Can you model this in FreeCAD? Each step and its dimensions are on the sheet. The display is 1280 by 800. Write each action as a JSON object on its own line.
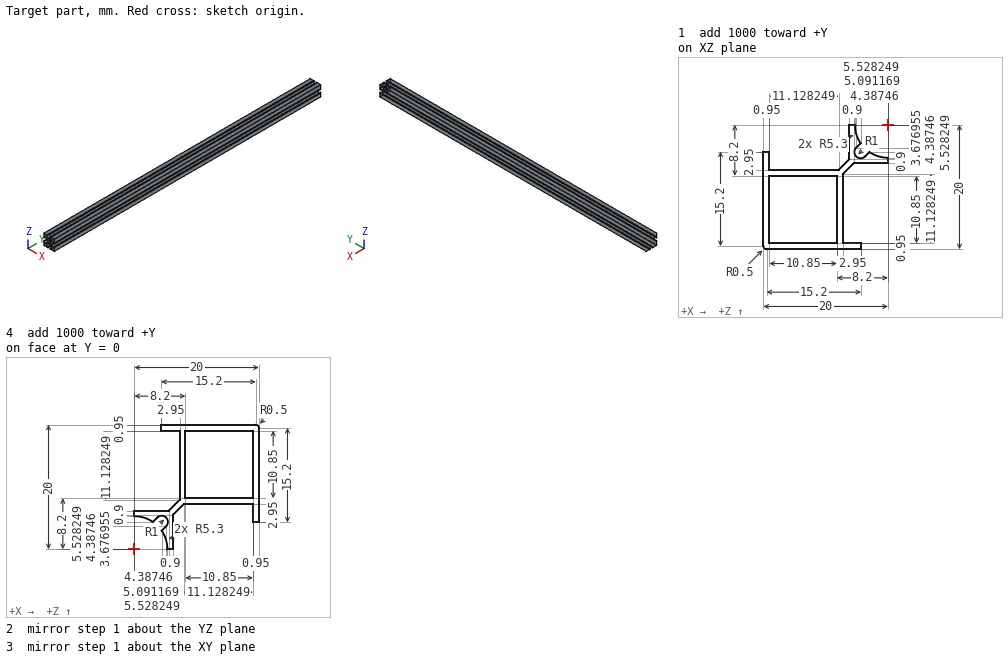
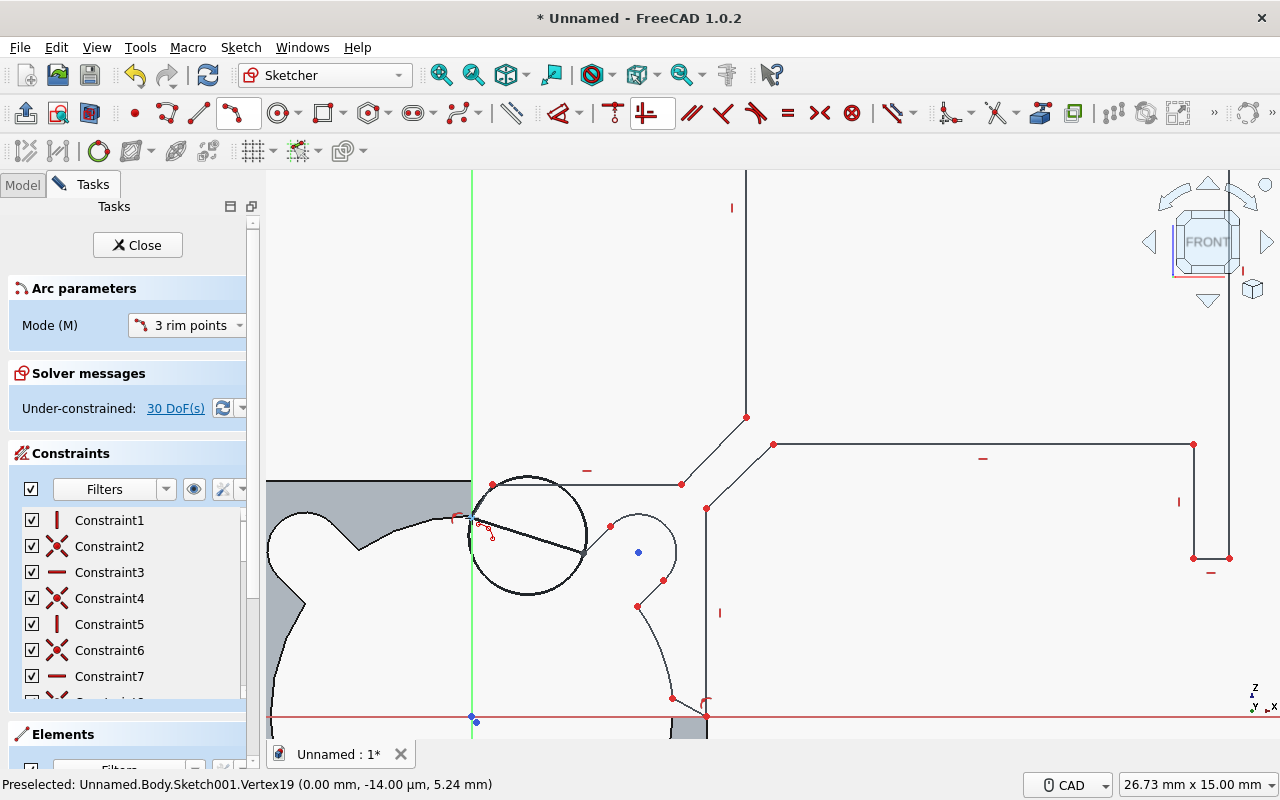
{"action": "scroll", "coordinate": [531, 524], "scroll_direction": "up", "scroll_amount": 3}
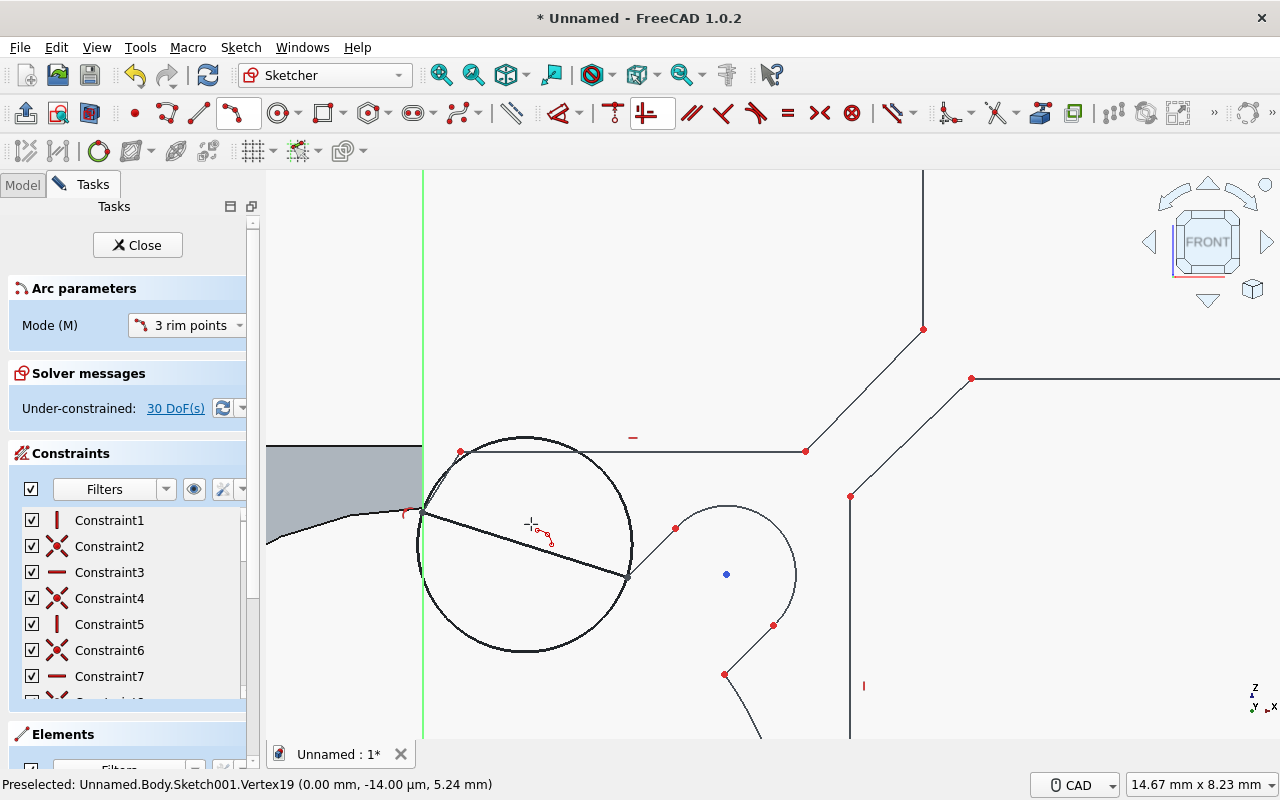
{"action": "left_click", "coordinate": [530, 524]}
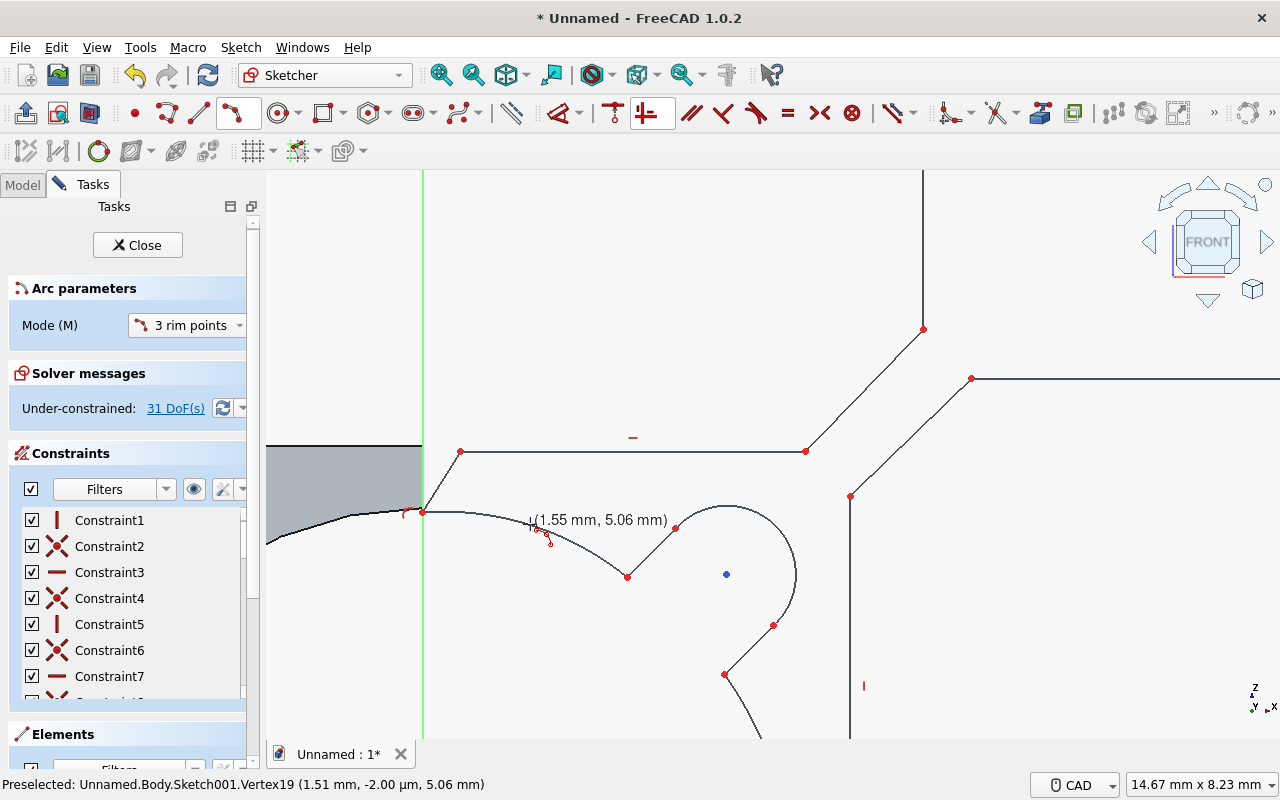
{"action": "scroll", "coordinate": [571, 543], "scroll_direction": "down", "scroll_amount": 7}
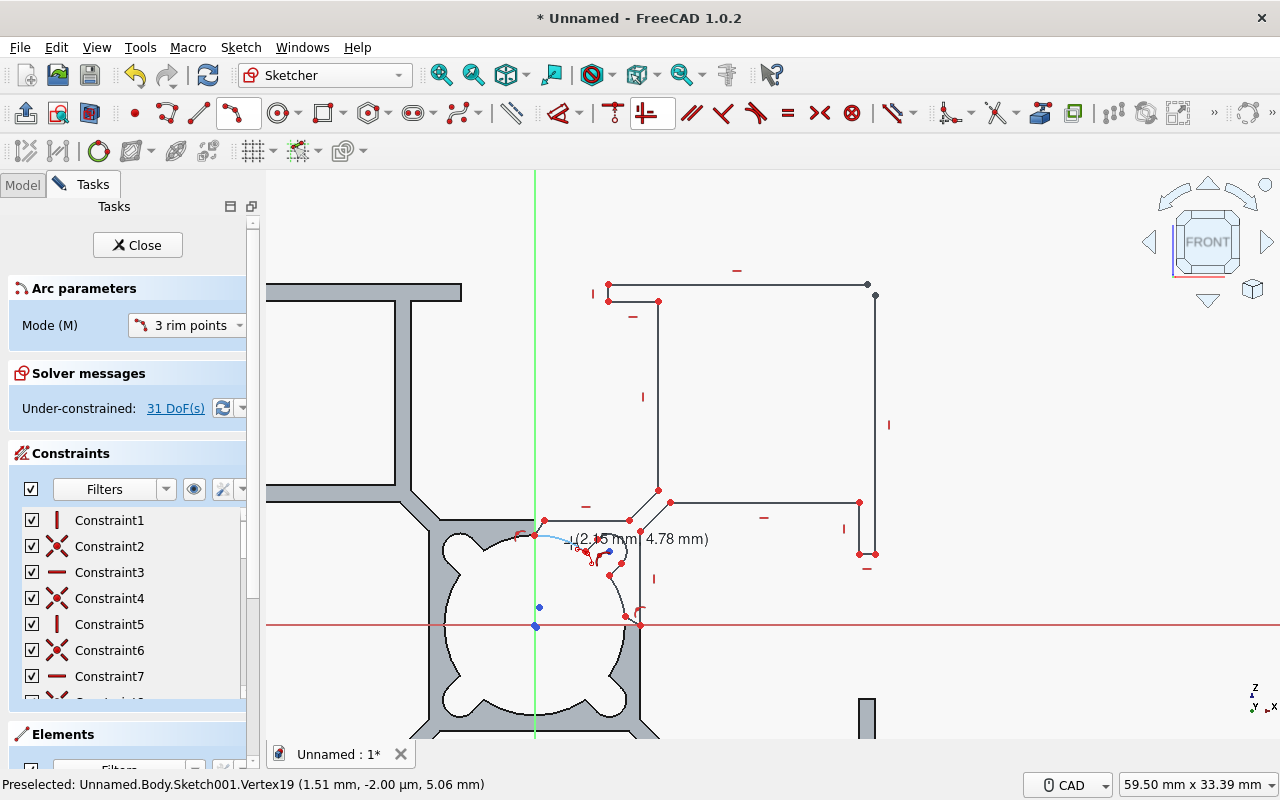
{"action": "scroll", "coordinate": [867, 284], "scroll_direction": "up", "scroll_amount": 2}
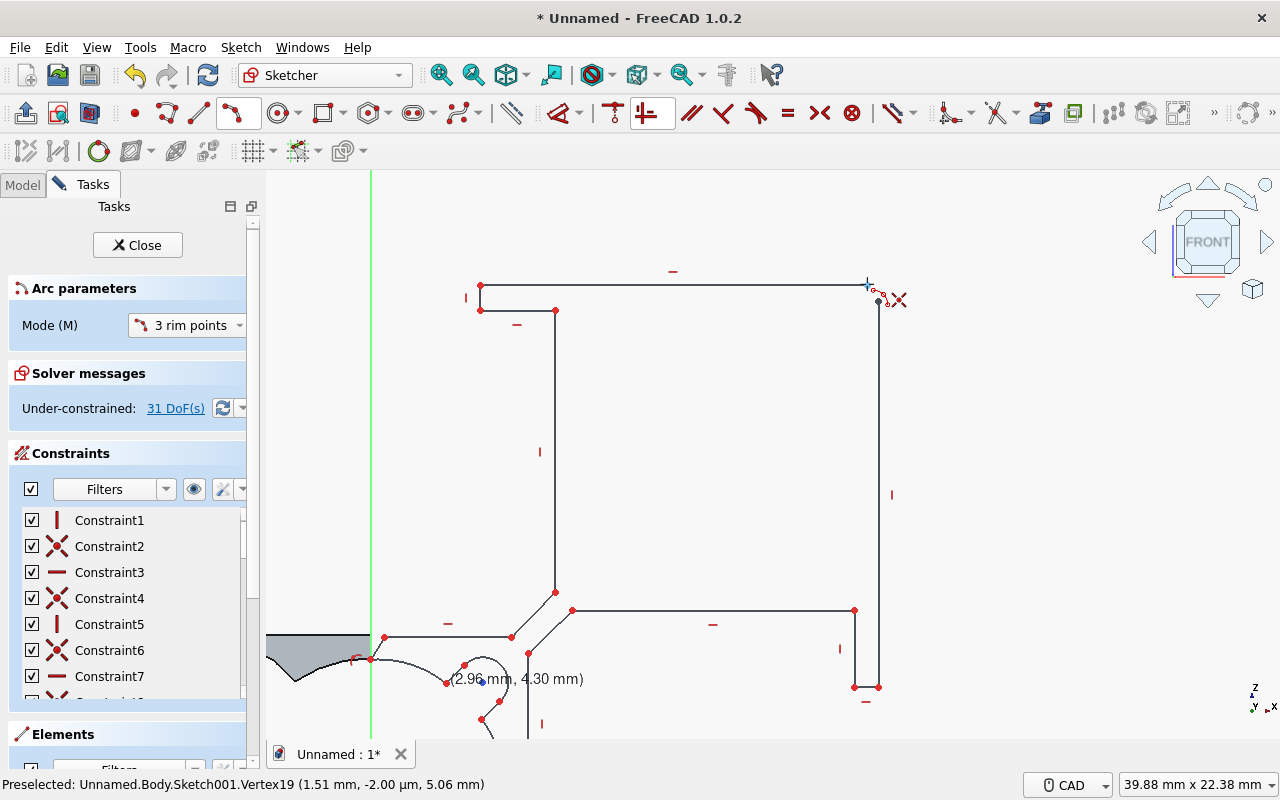
{"action": "left_click", "coordinate": [867, 285]}
{"action": "left_click", "coordinate": [879, 301]}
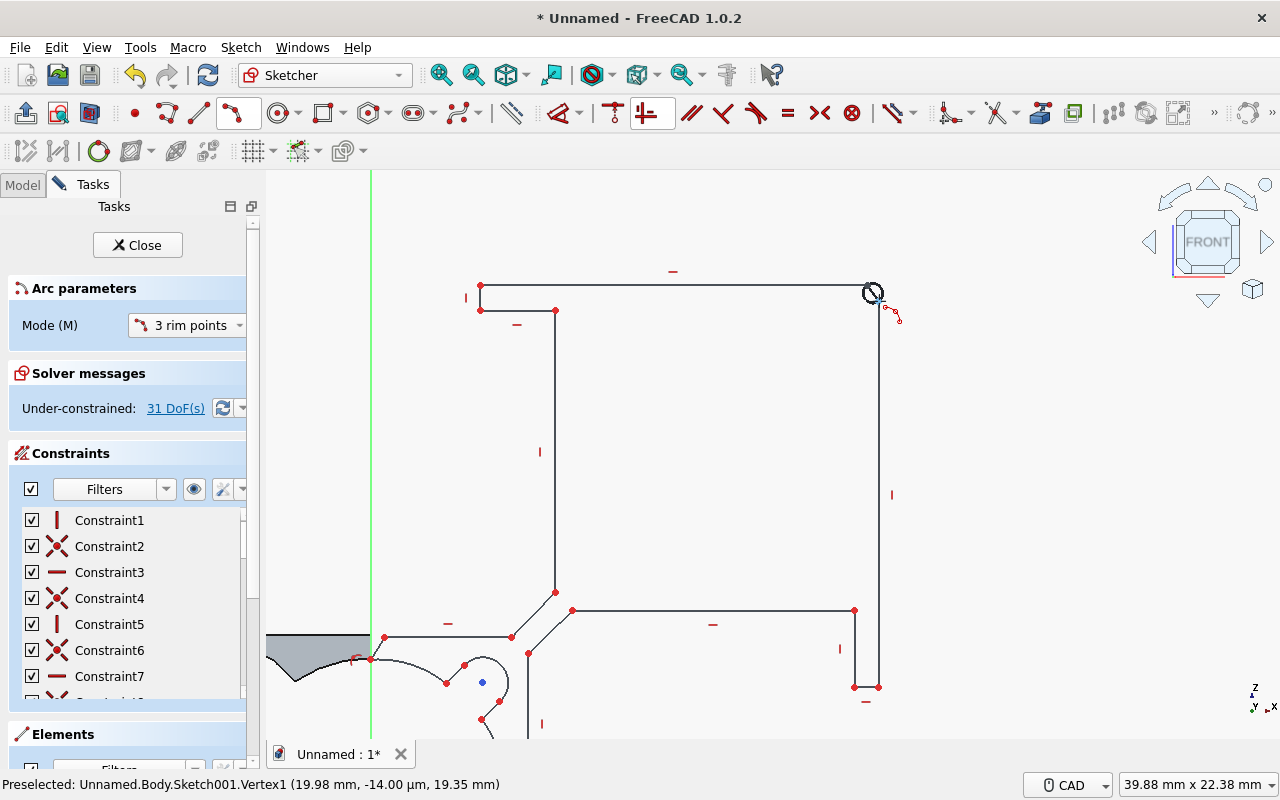
{"action": "scroll", "coordinate": [876, 288], "scroll_direction": "up", "scroll_amount": 8}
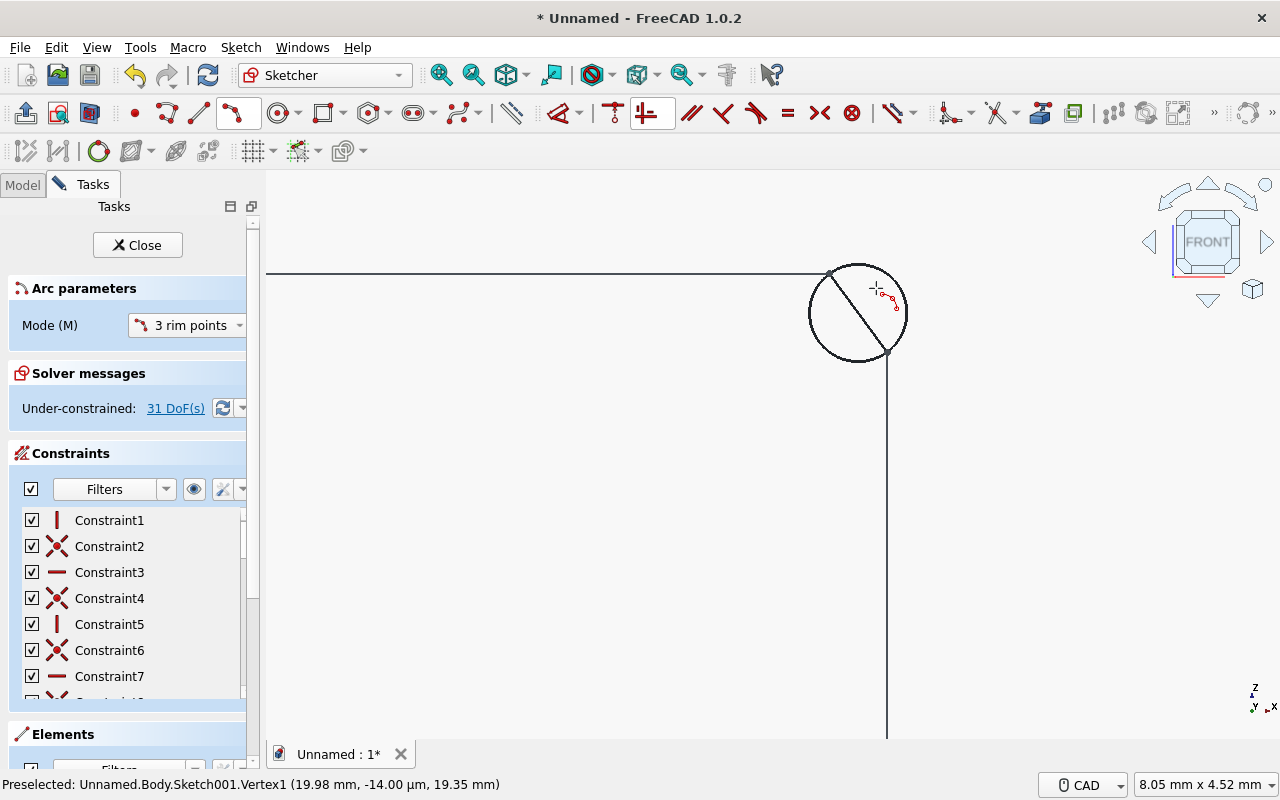
{"action": "left_click", "coordinate": [872, 288]}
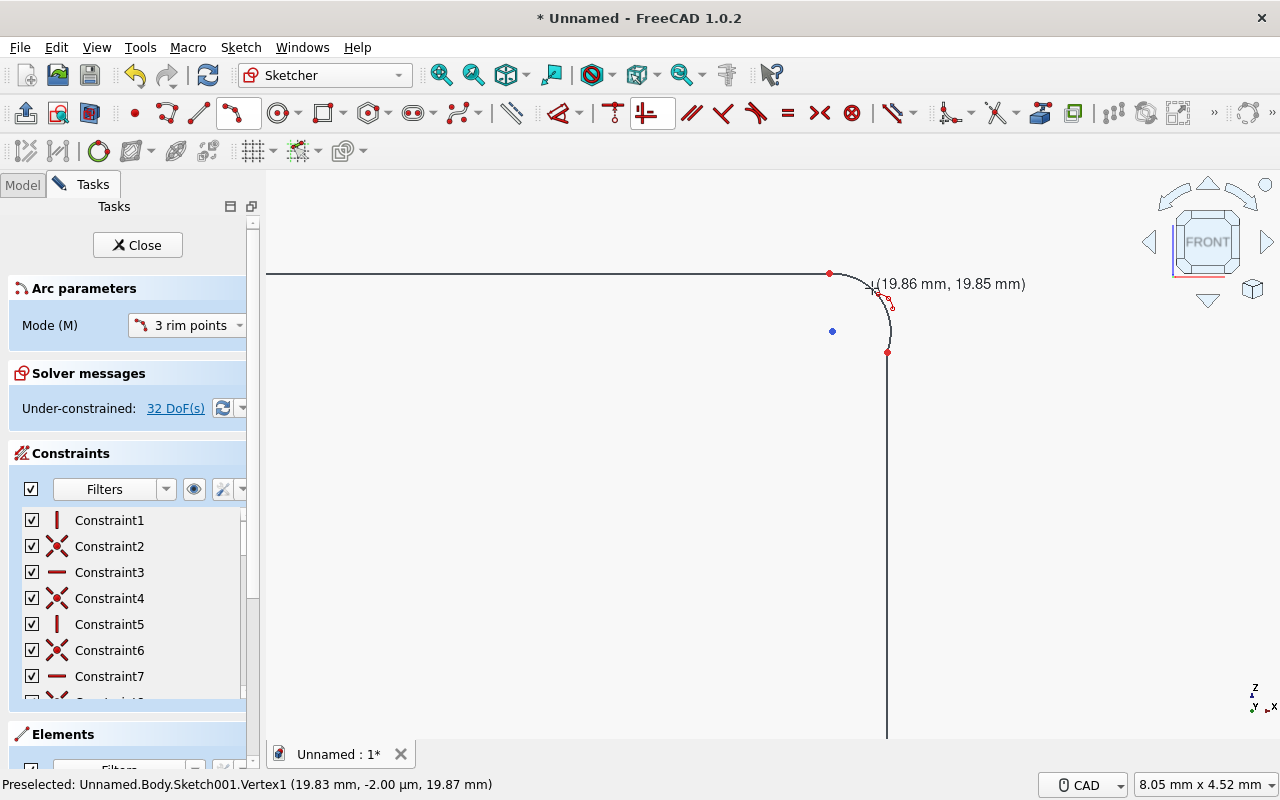
{"action": "key", "text": "g r"}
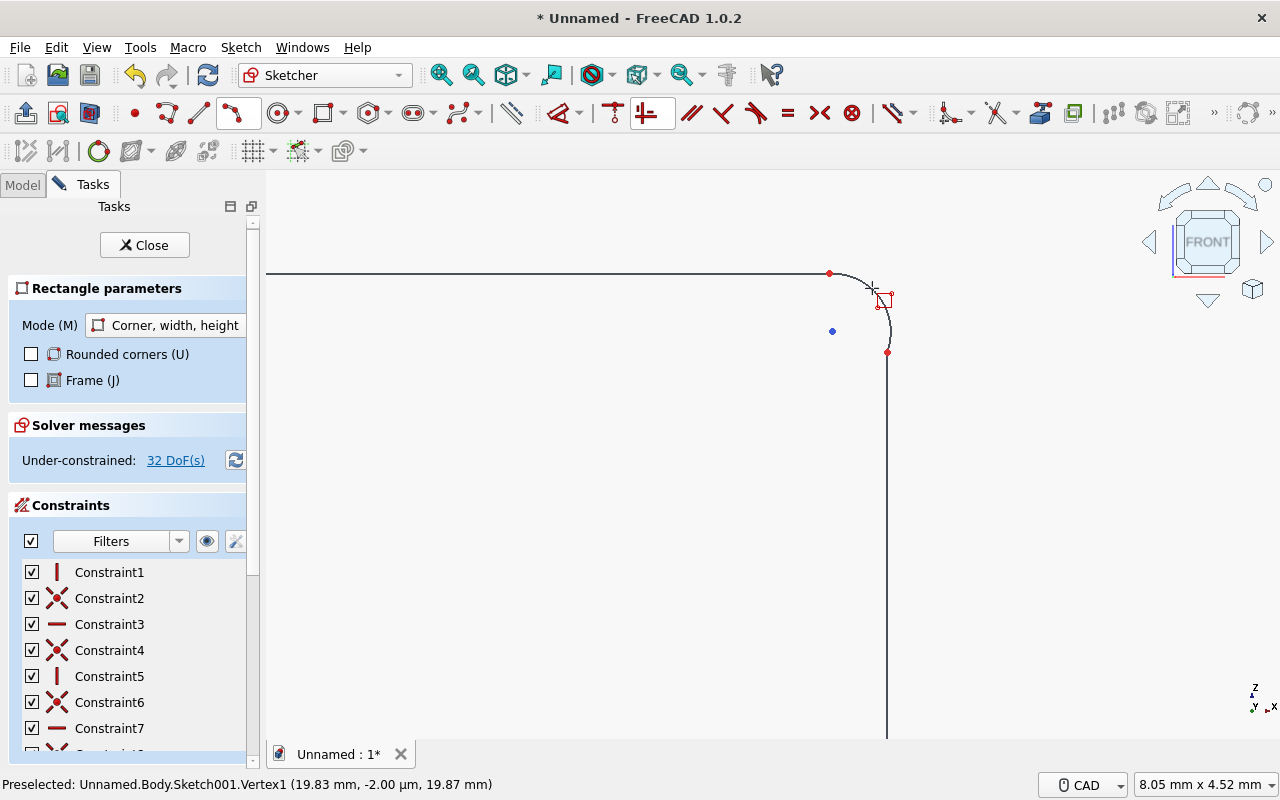
{"action": "scroll", "coordinate": [873, 286], "scroll_direction": "down", "scroll_amount": 10}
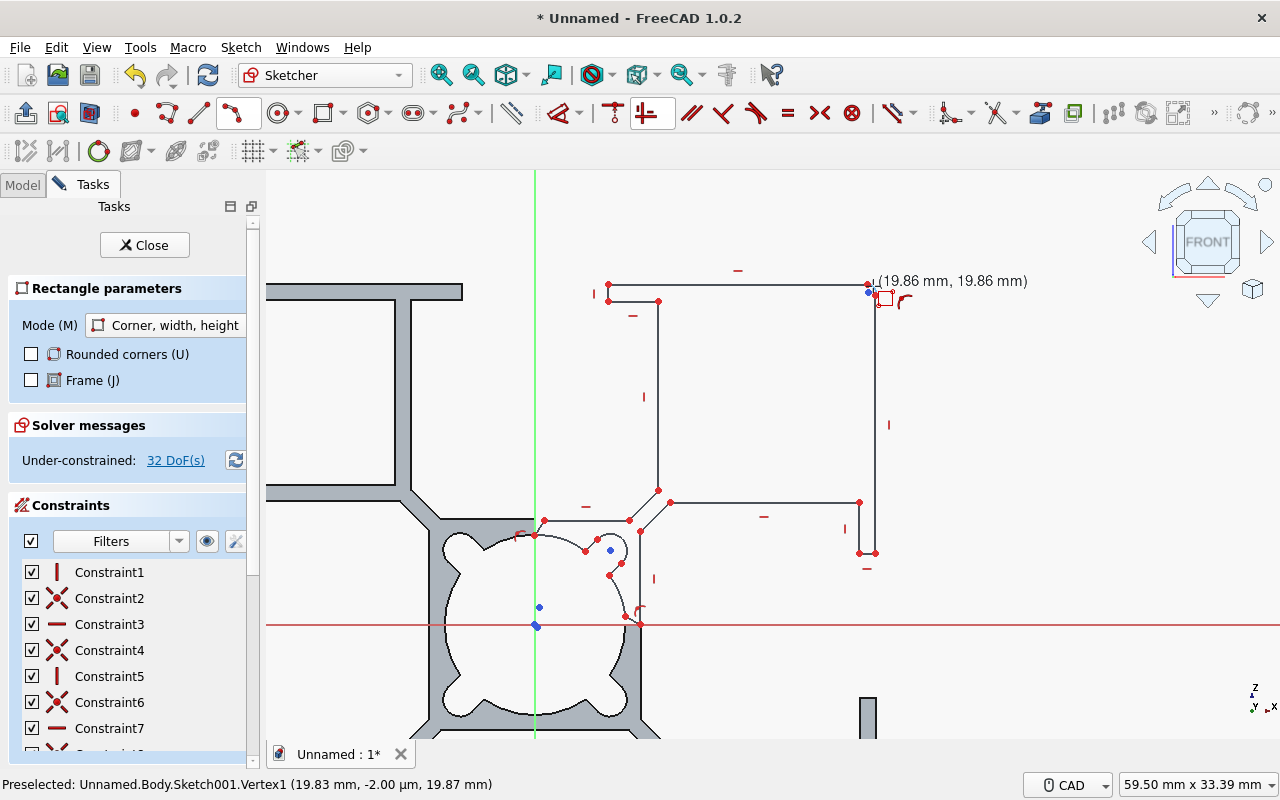
{"action": "left_click", "coordinate": [675, 300]}
{"action": "mouse_move", "coordinate": [860, 485]}